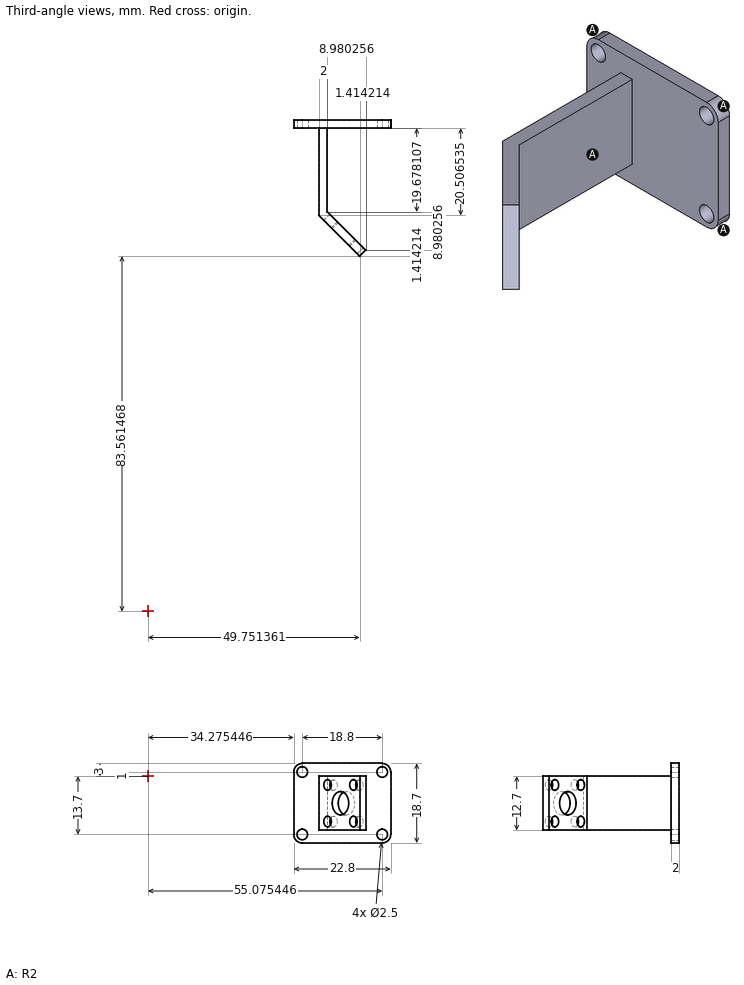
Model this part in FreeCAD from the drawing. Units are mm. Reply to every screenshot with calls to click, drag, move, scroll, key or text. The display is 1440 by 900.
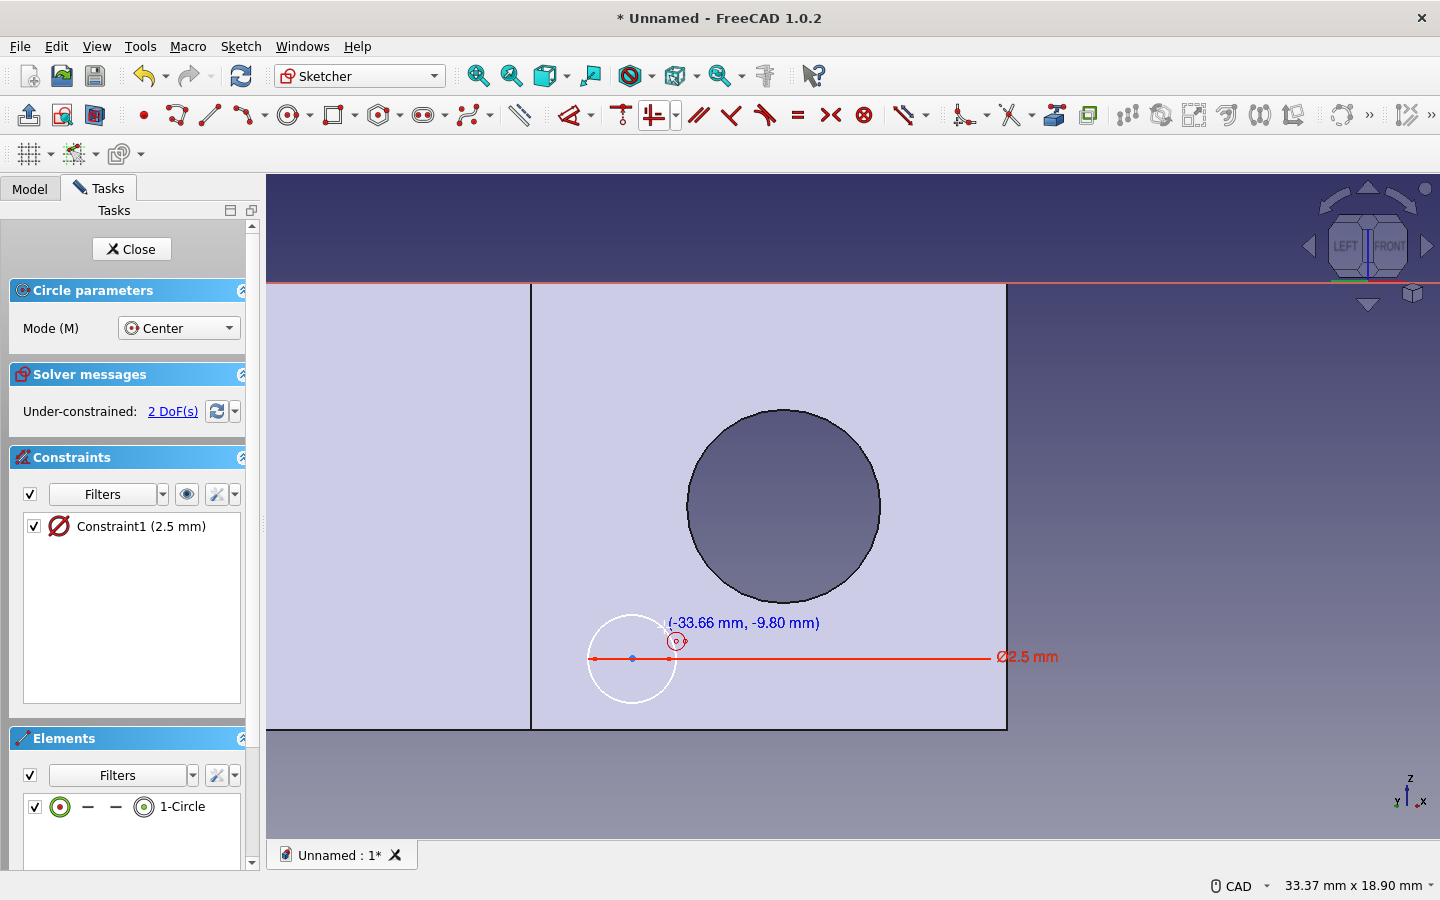
click(632, 355)
move(664, 324)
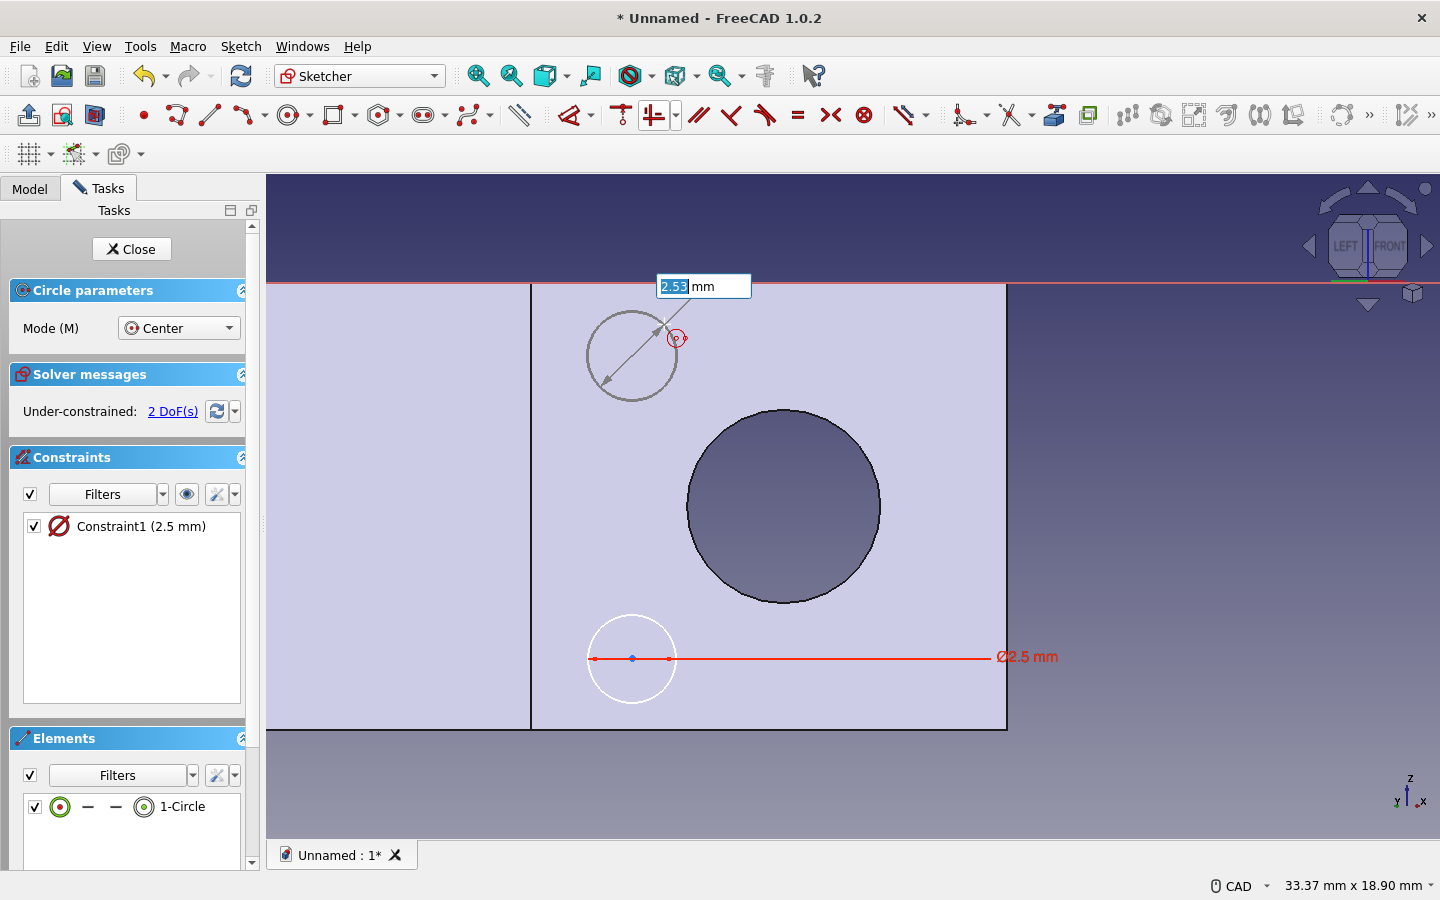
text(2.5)
key(Return)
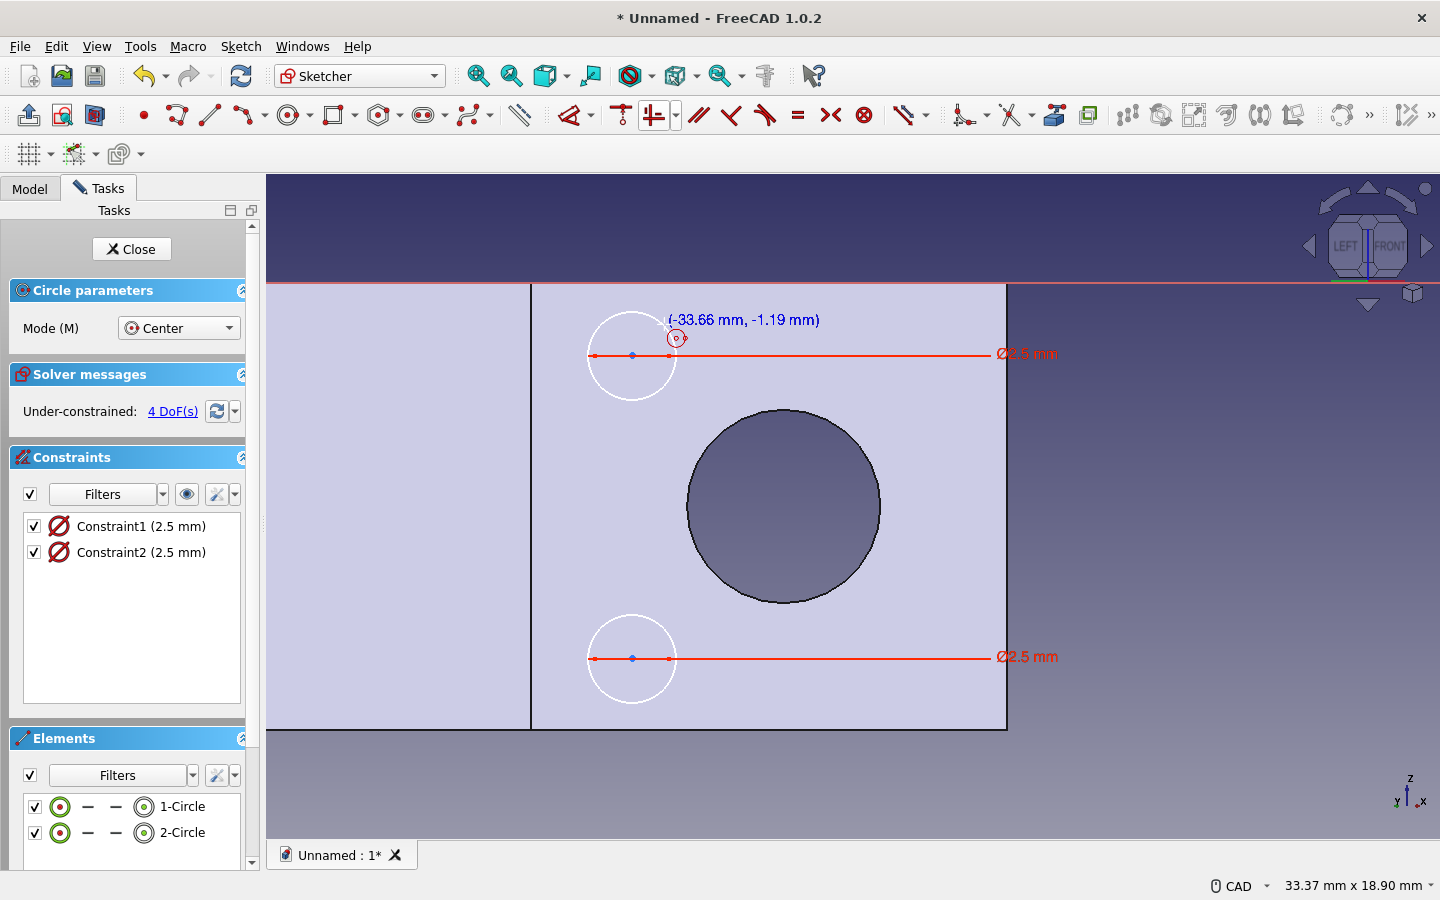
click(935, 355)
move(966, 324)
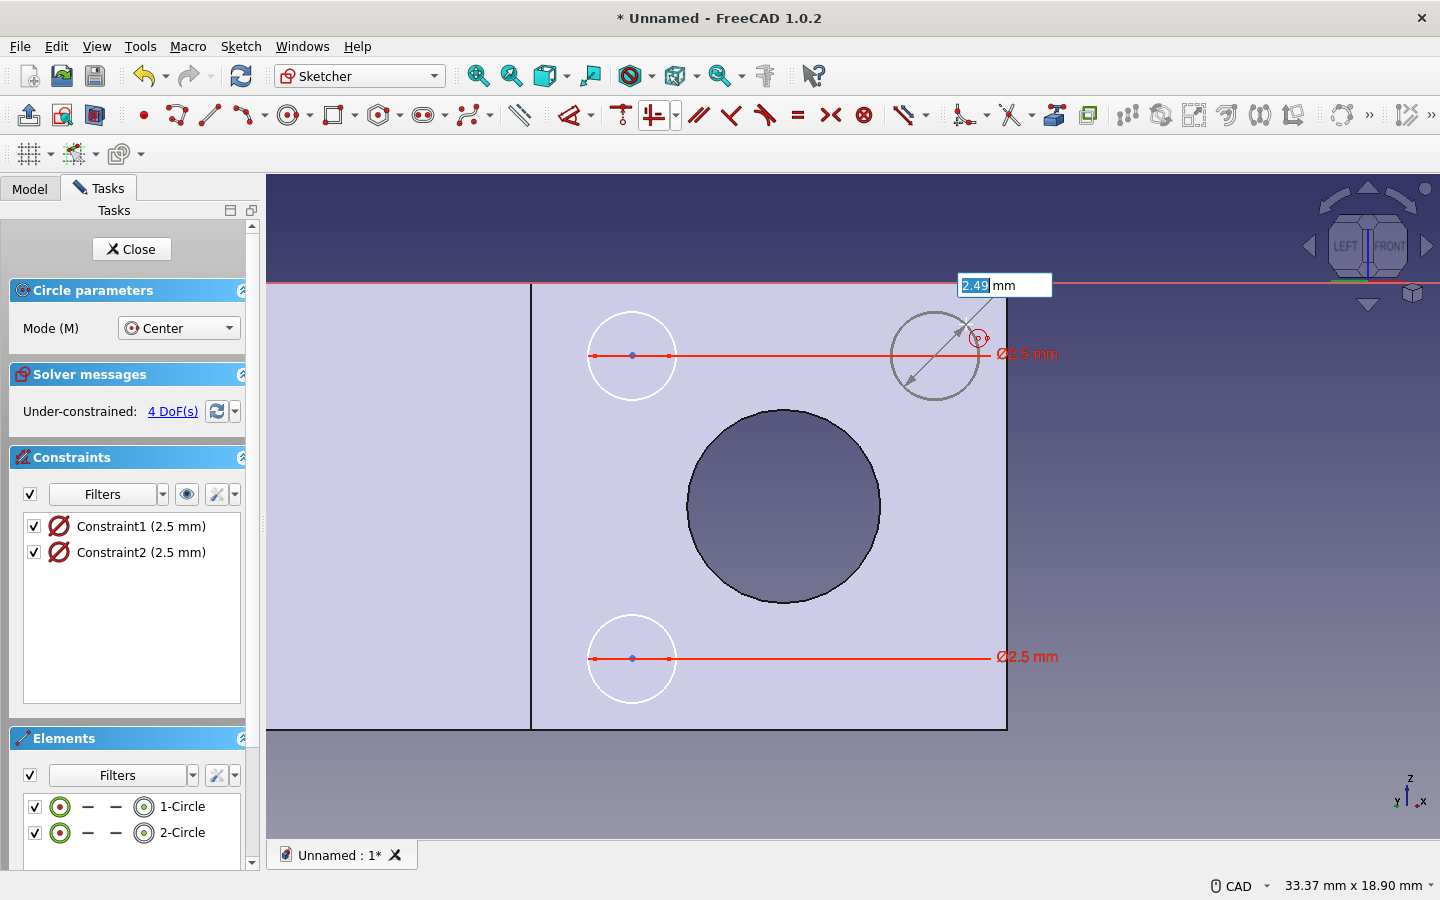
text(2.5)
key(Return)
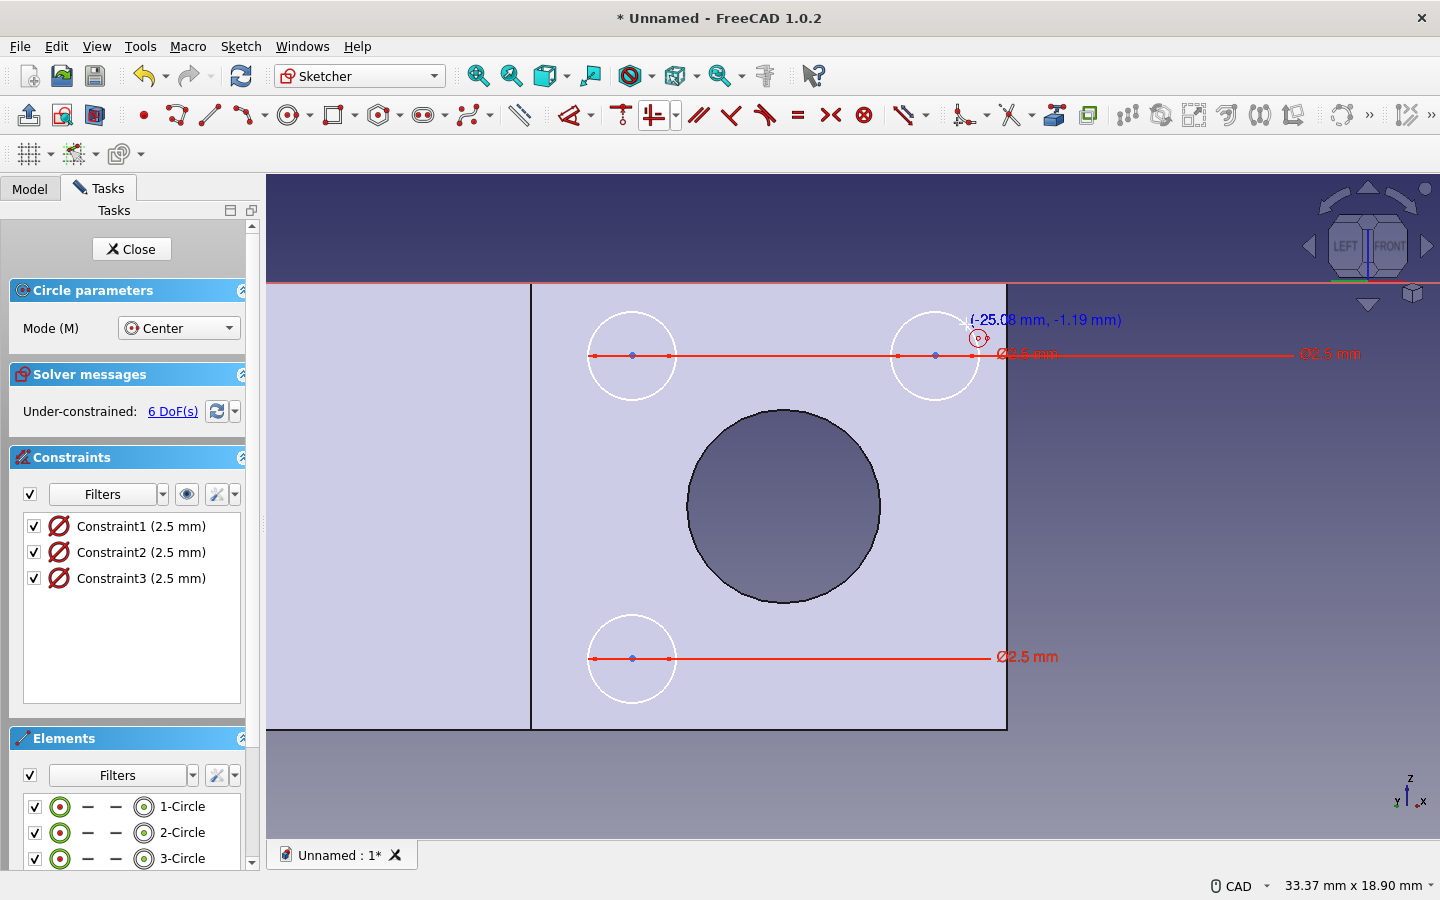
click(935, 658)
move(966, 627)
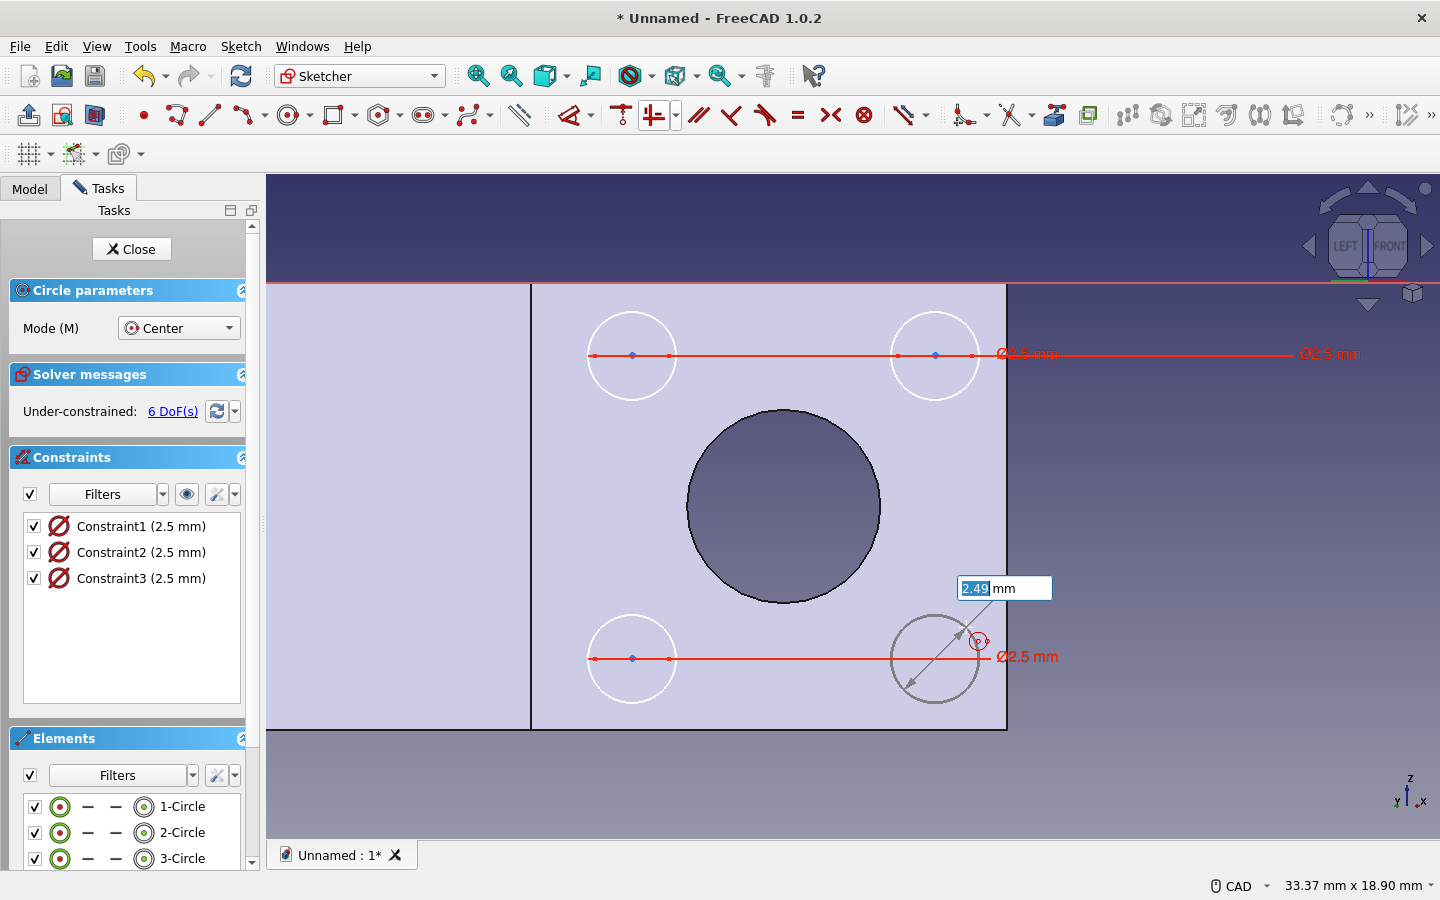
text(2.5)
key(Return)
key(Escape)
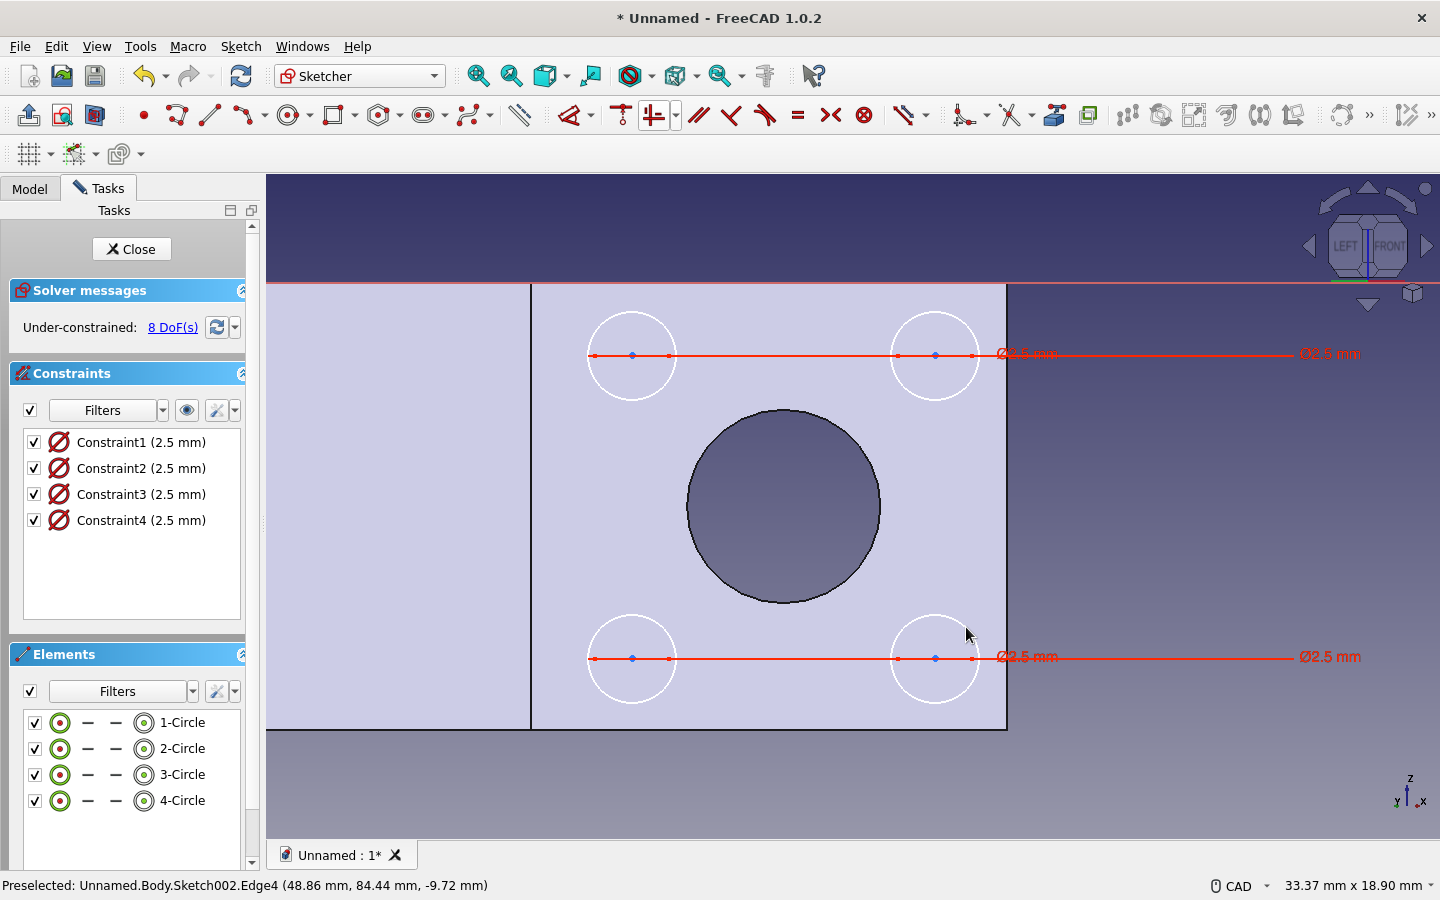
key(d)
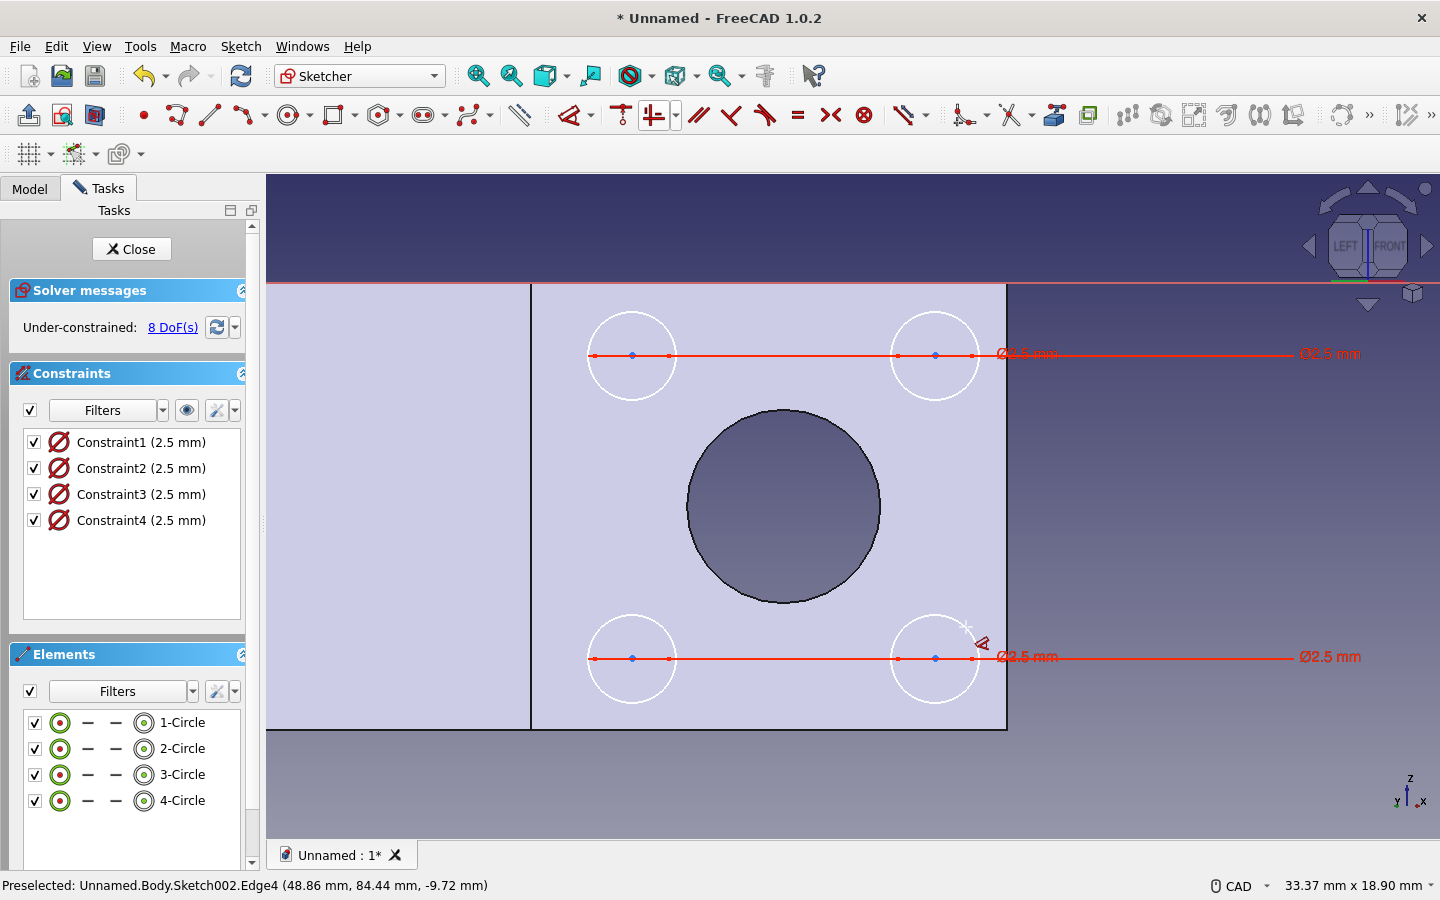
click(632, 356)
click(598, 303)